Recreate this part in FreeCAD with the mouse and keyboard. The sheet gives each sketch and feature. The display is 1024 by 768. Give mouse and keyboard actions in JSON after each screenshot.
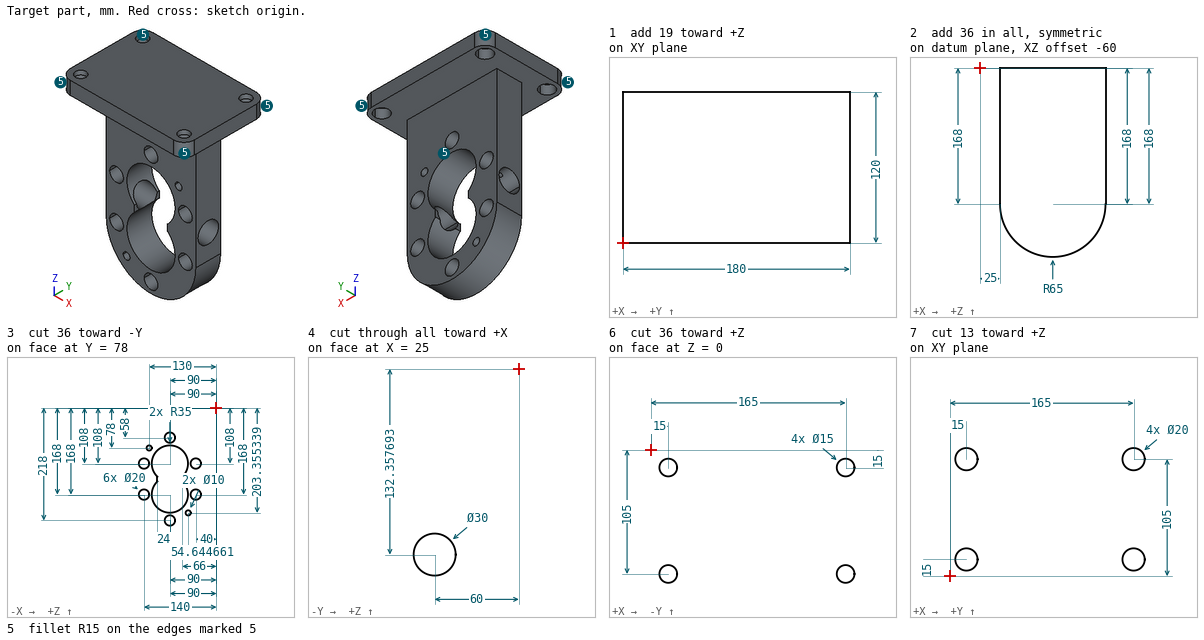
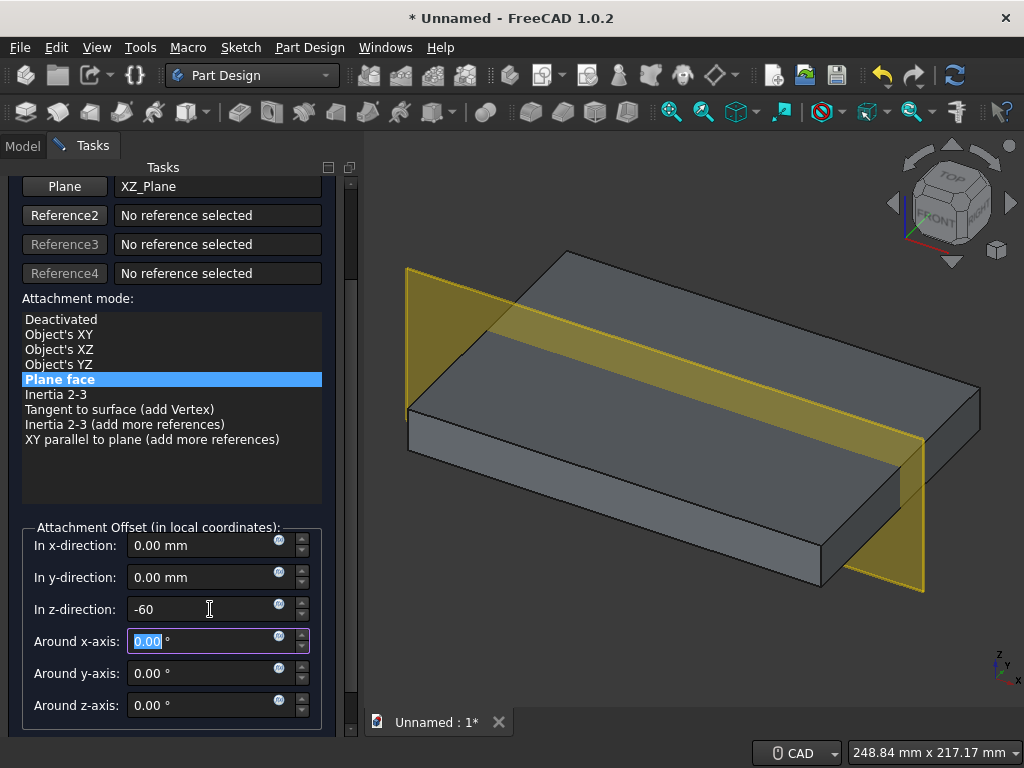
{"action": "scroll", "coordinate": [351, 456], "scroll_direction": "up", "scroll_amount": 3}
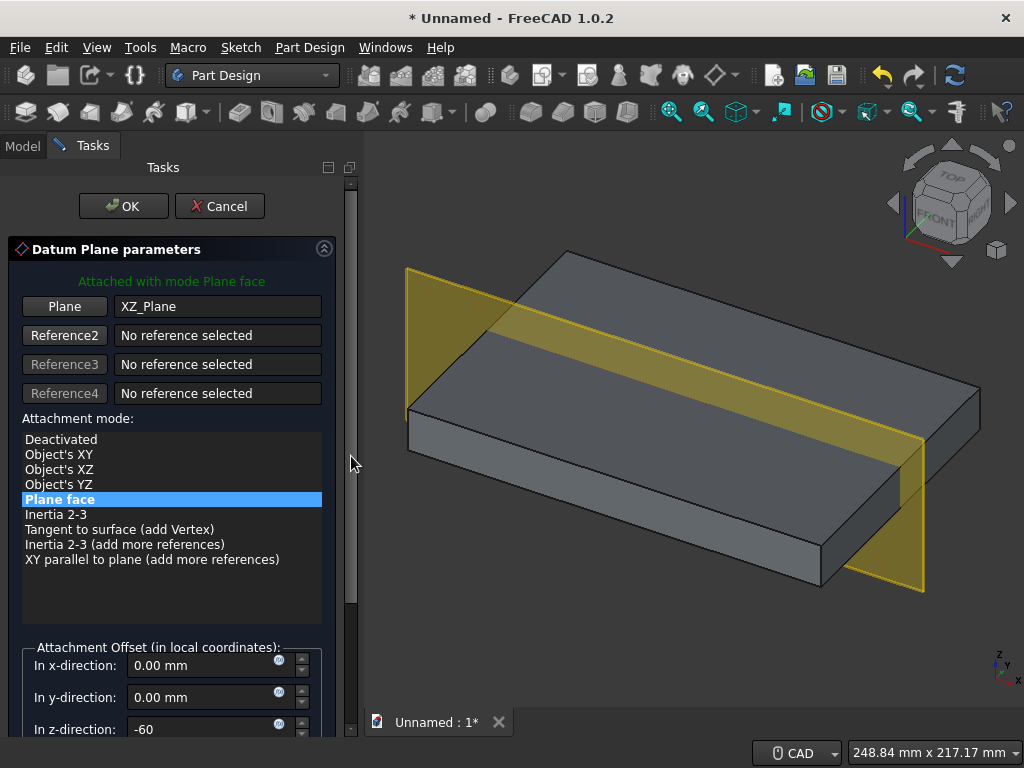
{"action": "left_click", "coordinate": [124, 206]}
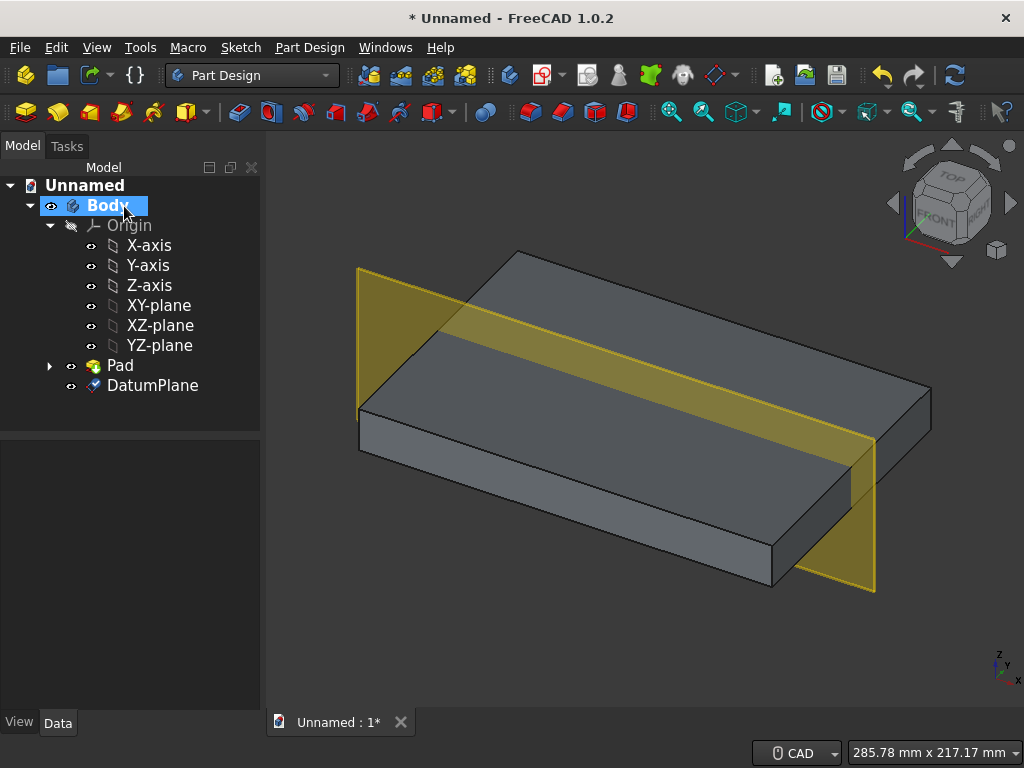
{"action": "left_click", "coordinate": [116, 386]}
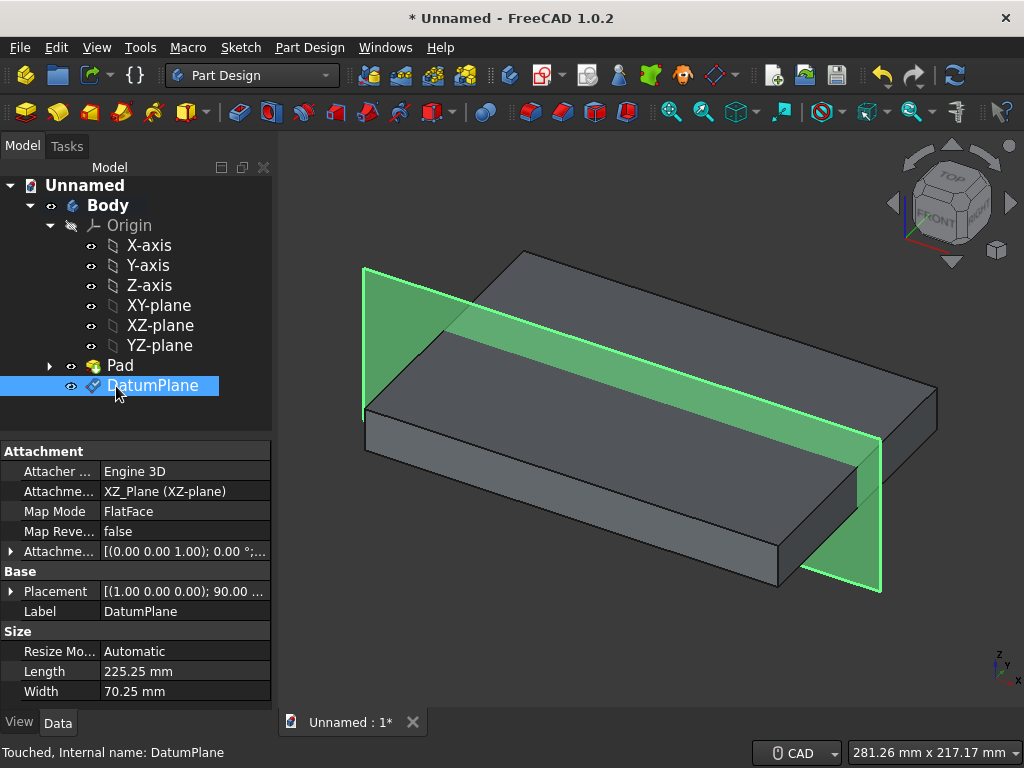
{"action": "left_click", "coordinate": [542, 76]}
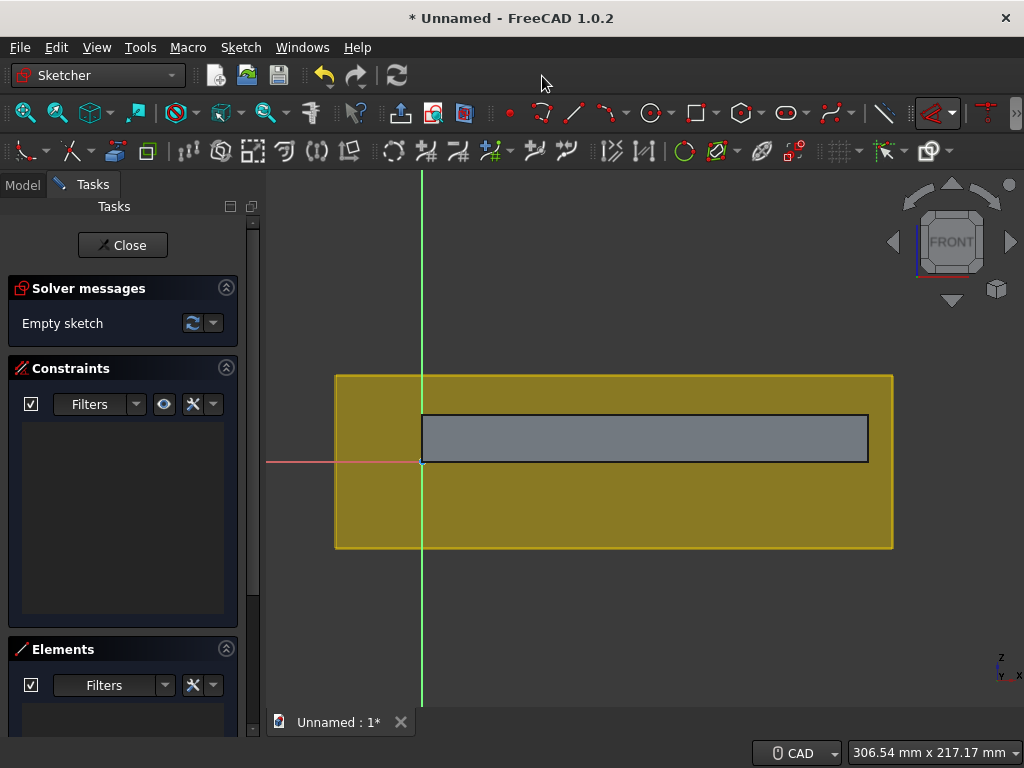
{"action": "left_click", "coordinate": [466, 114]}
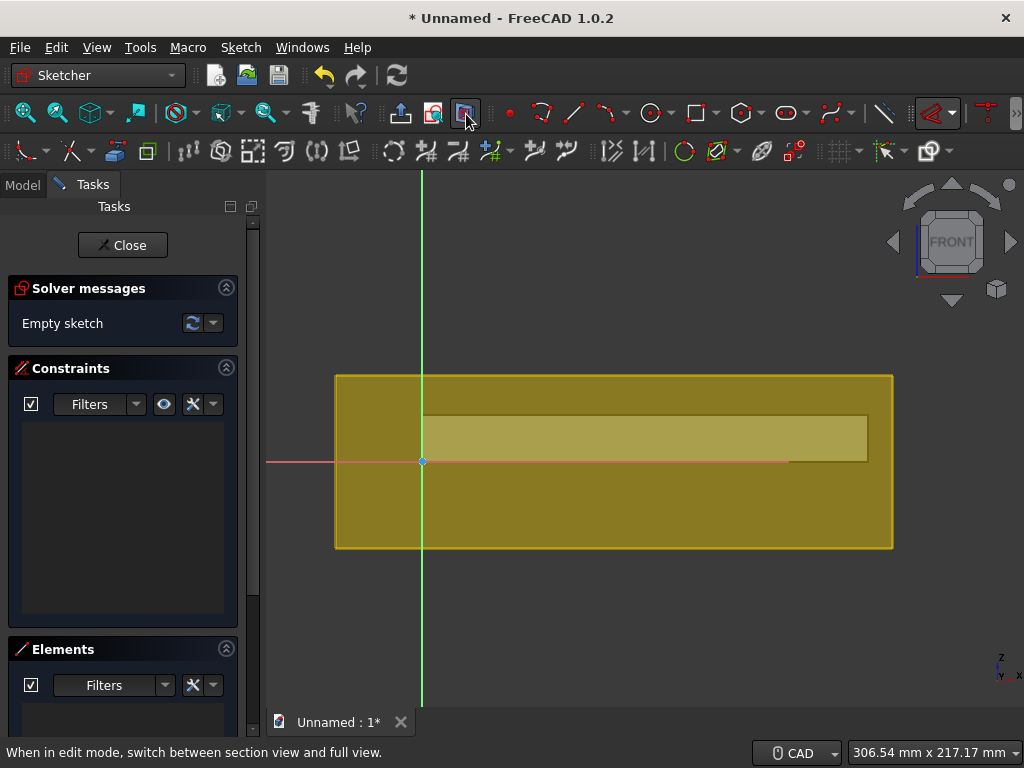
{"action": "scroll", "coordinate": [546, 198], "scroll_direction": "down", "scroll_amount": 4}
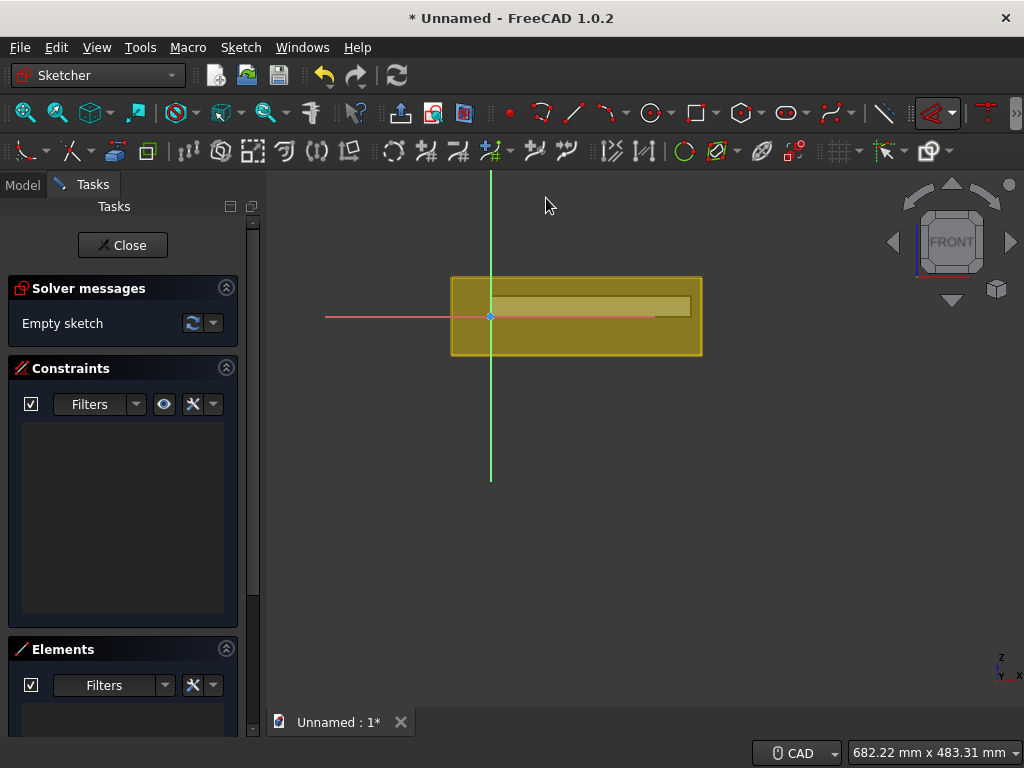
{"action": "left_click", "coordinate": [542, 114]}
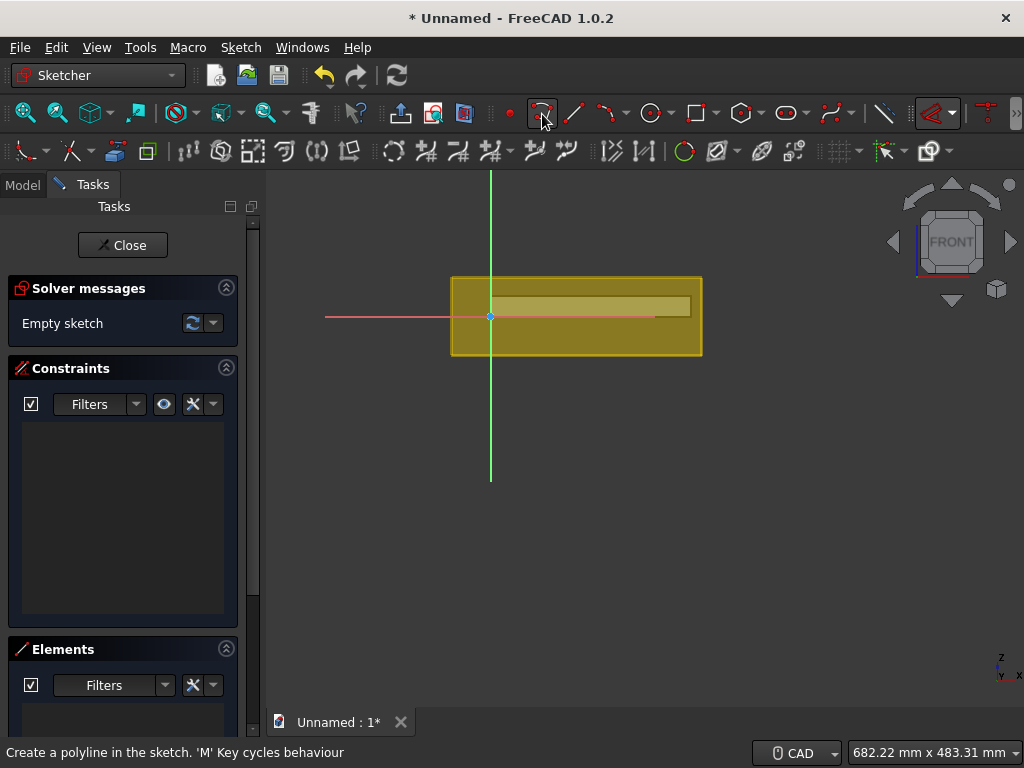
{"action": "left_click", "coordinate": [518, 503]}
{"action": "left_click", "coordinate": [518, 317]}
{"action": "left_click", "coordinate": [663, 326]}
{"action": "left_click", "coordinate": [663, 503]}
{"action": "right_click", "coordinate": [663, 503]}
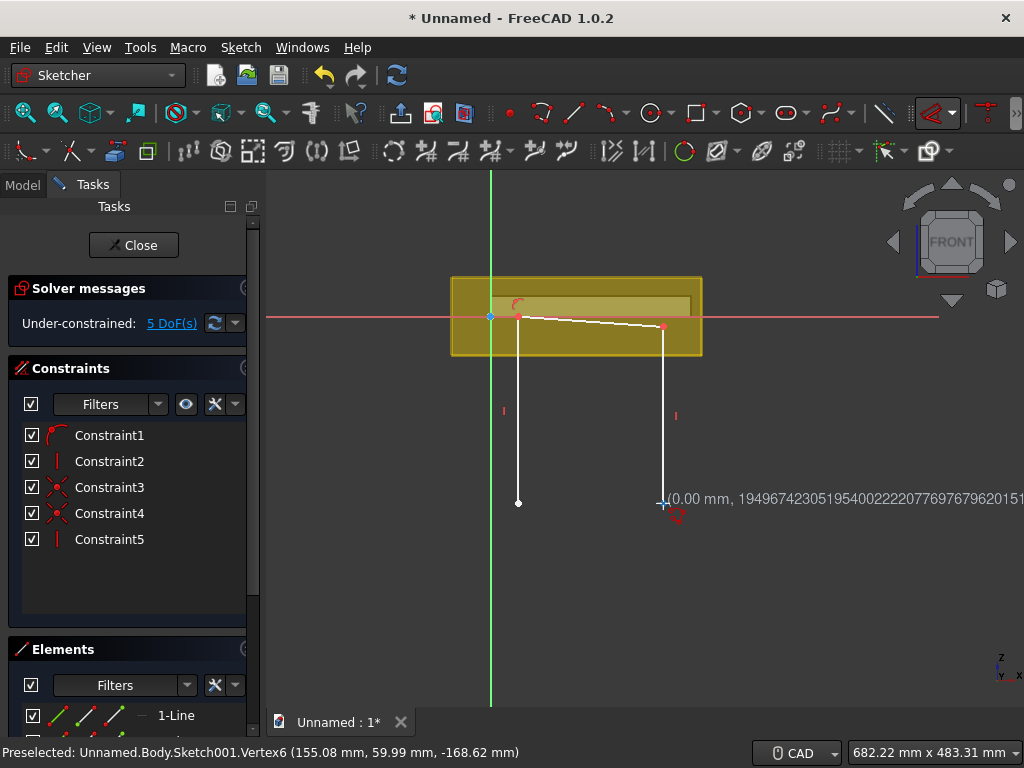
{"action": "left_click", "coordinate": [606, 114]}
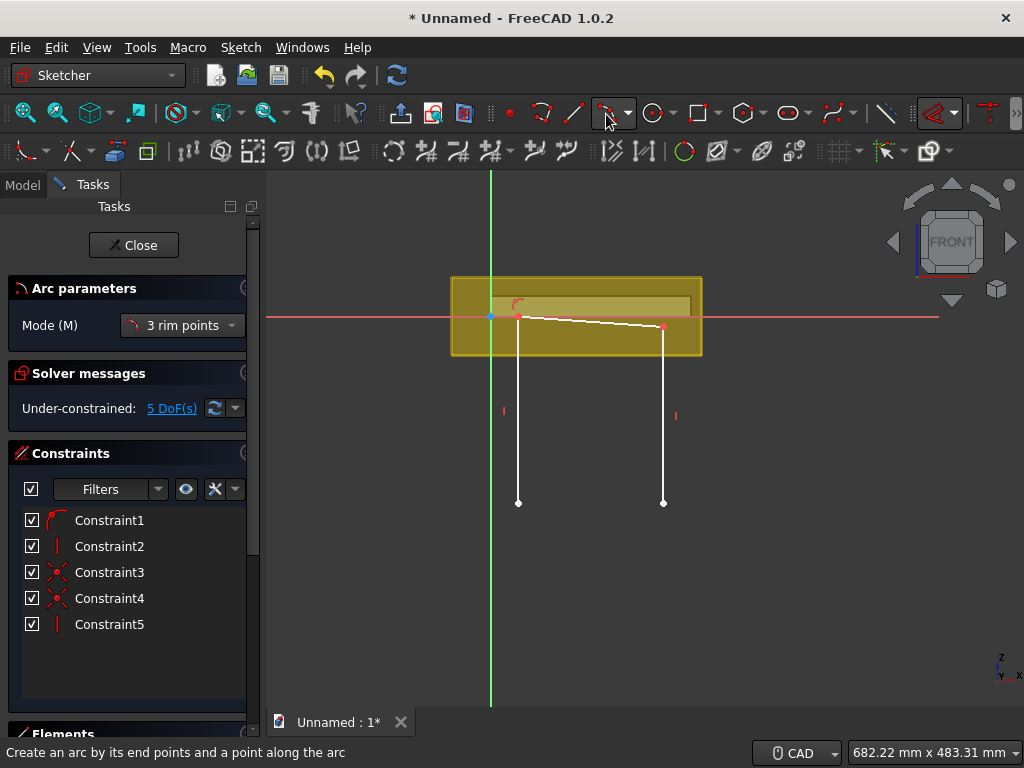
{"action": "left_click", "coordinate": [663, 504]}
{"action": "left_click", "coordinate": [518, 504]}
{"action": "left_click", "coordinate": [591, 576]}
{"action": "key", "text": "Escape"}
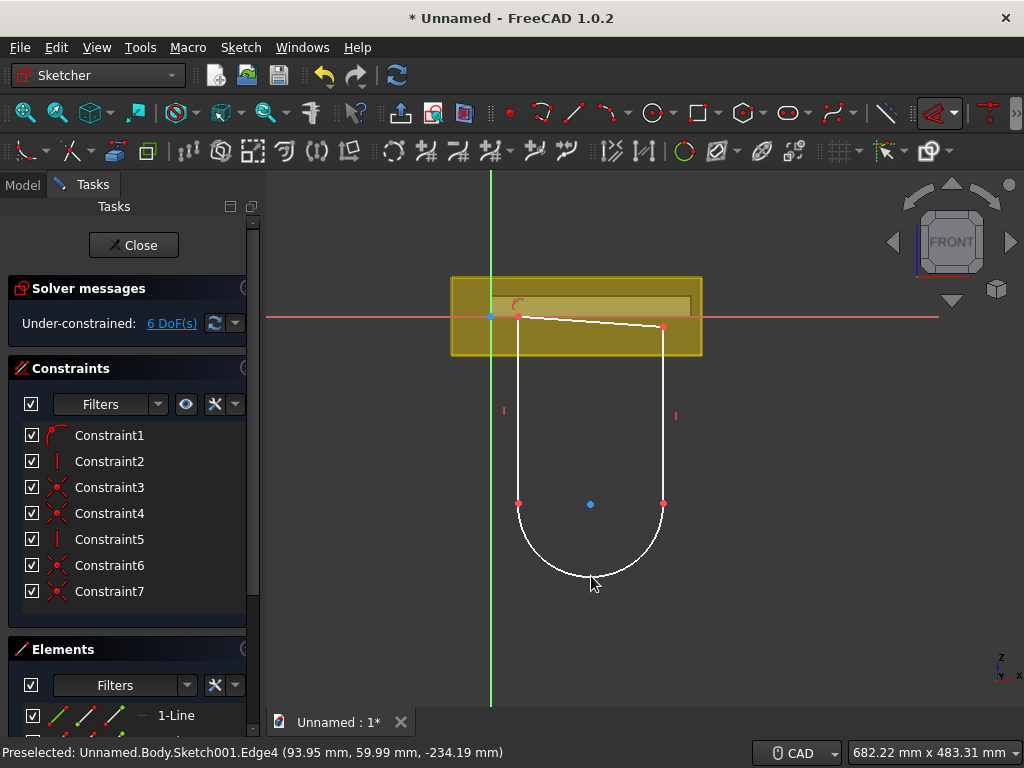
{"action": "left_click", "coordinate": [562, 320]}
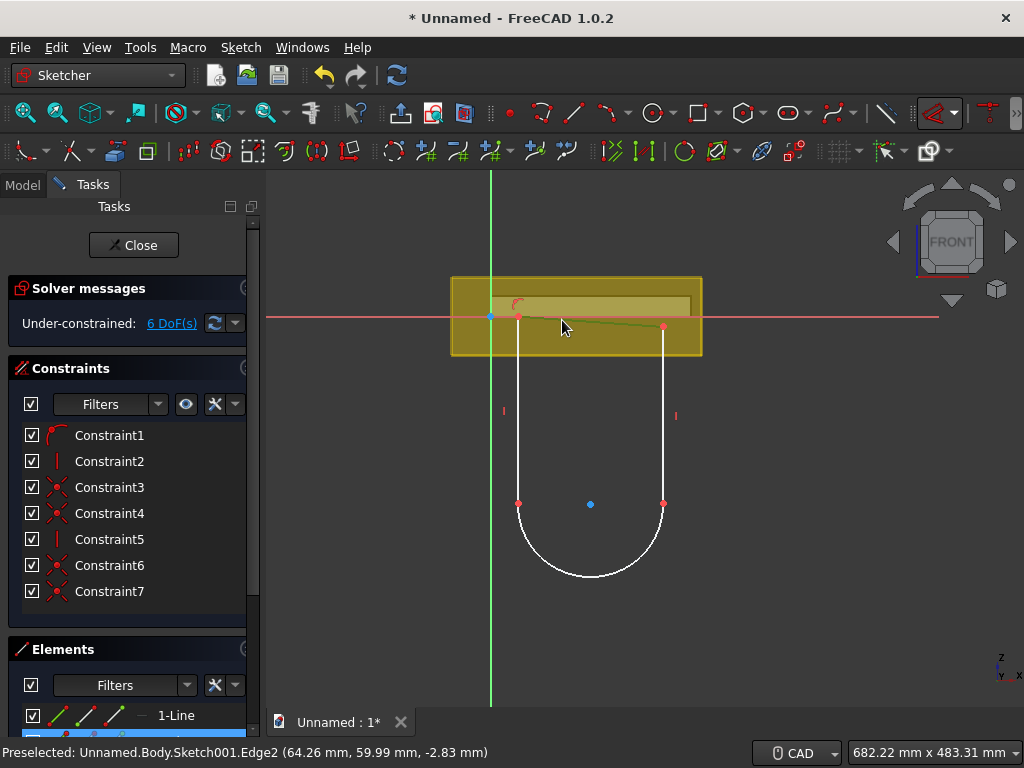
{"action": "key", "text": "h"}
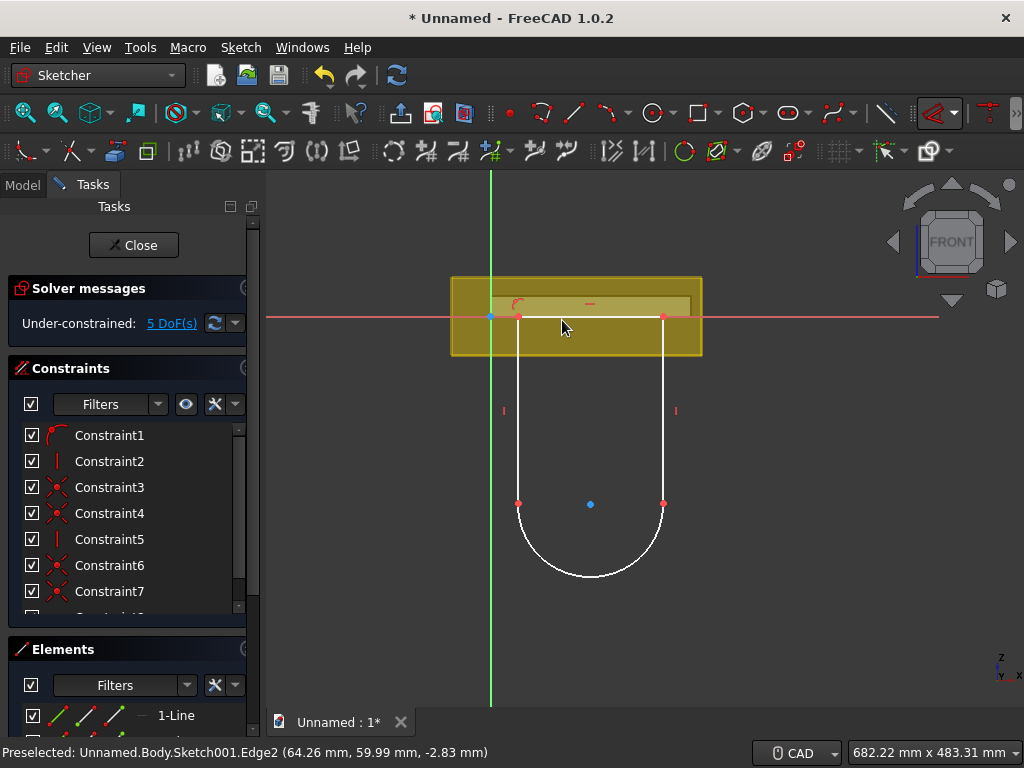
{"action": "left_click", "coordinate": [548, 563]}